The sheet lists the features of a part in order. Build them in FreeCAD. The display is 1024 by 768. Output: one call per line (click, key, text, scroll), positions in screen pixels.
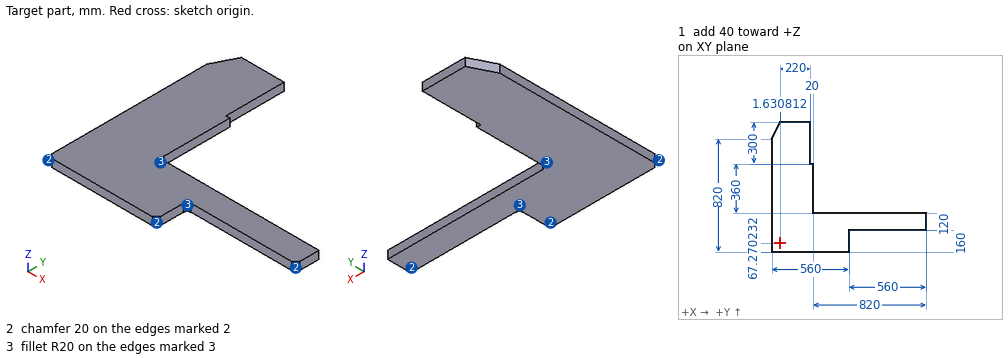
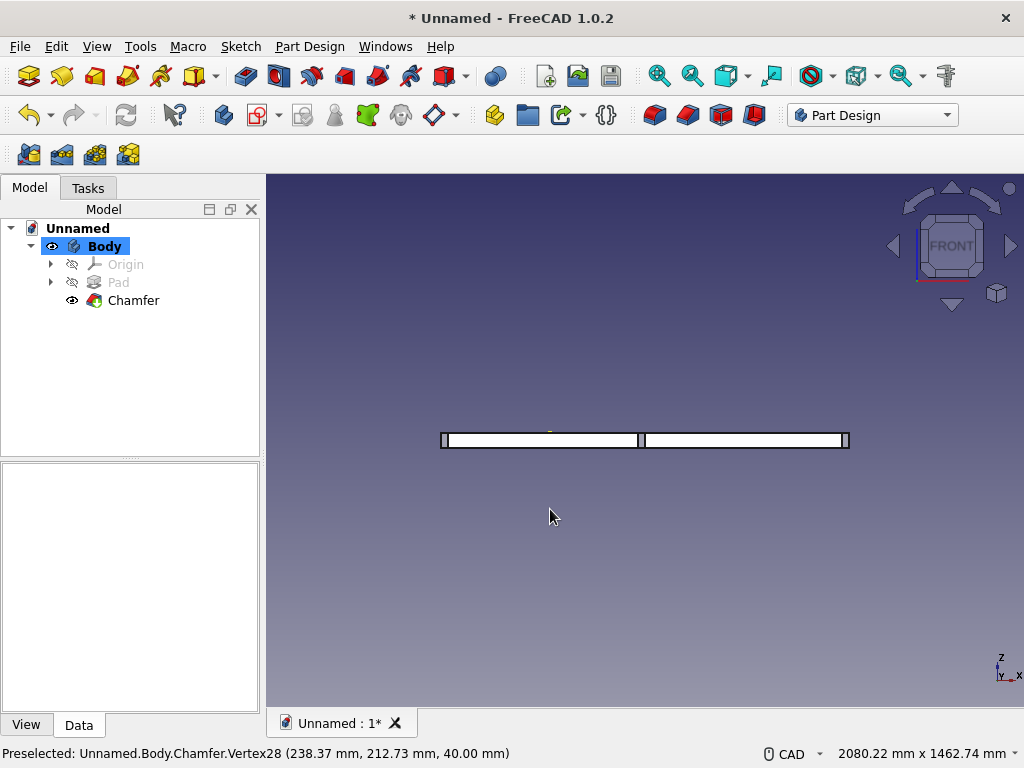
scroll(550, 439, up, 6)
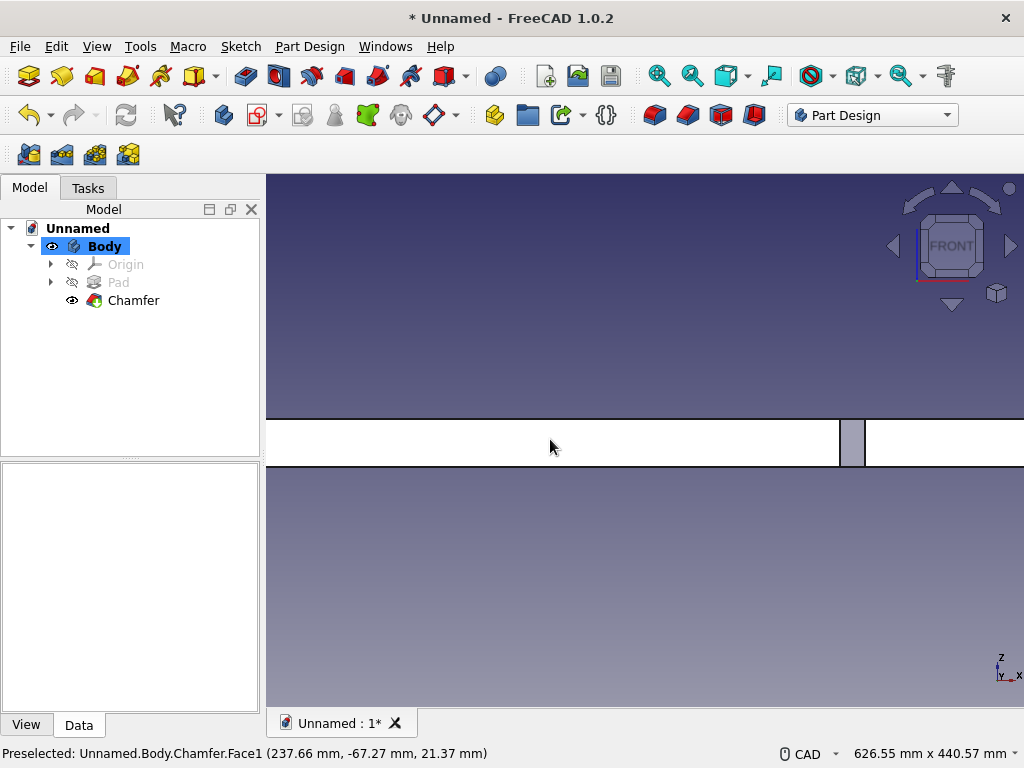
key(v)
key(f)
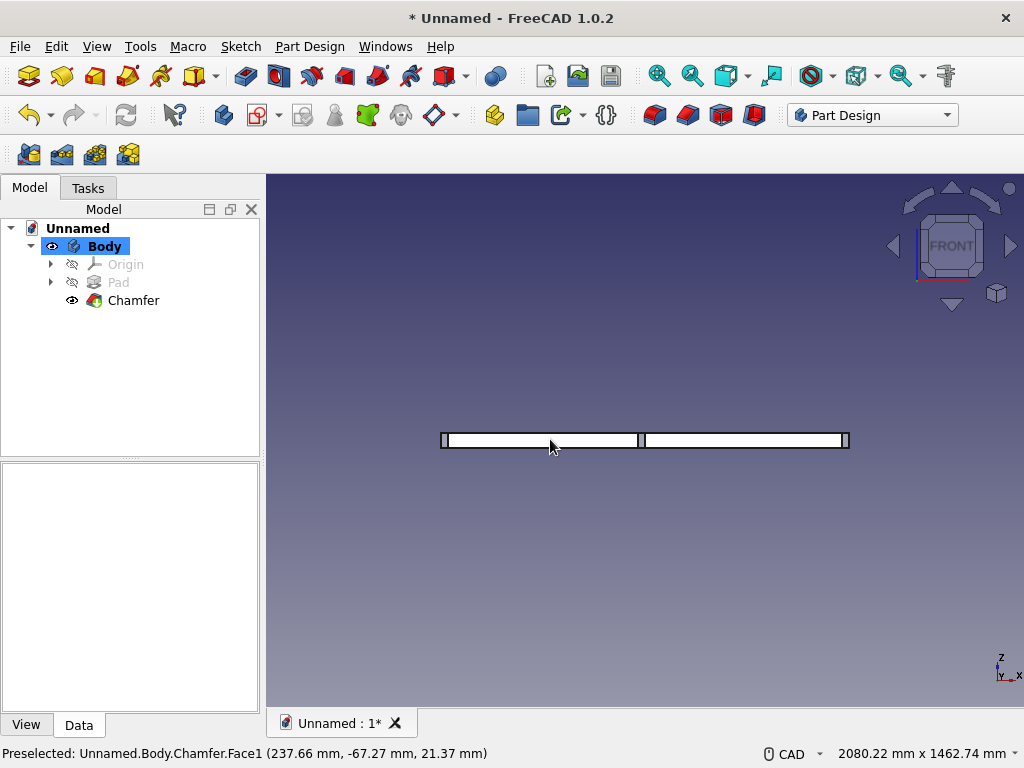
key(3)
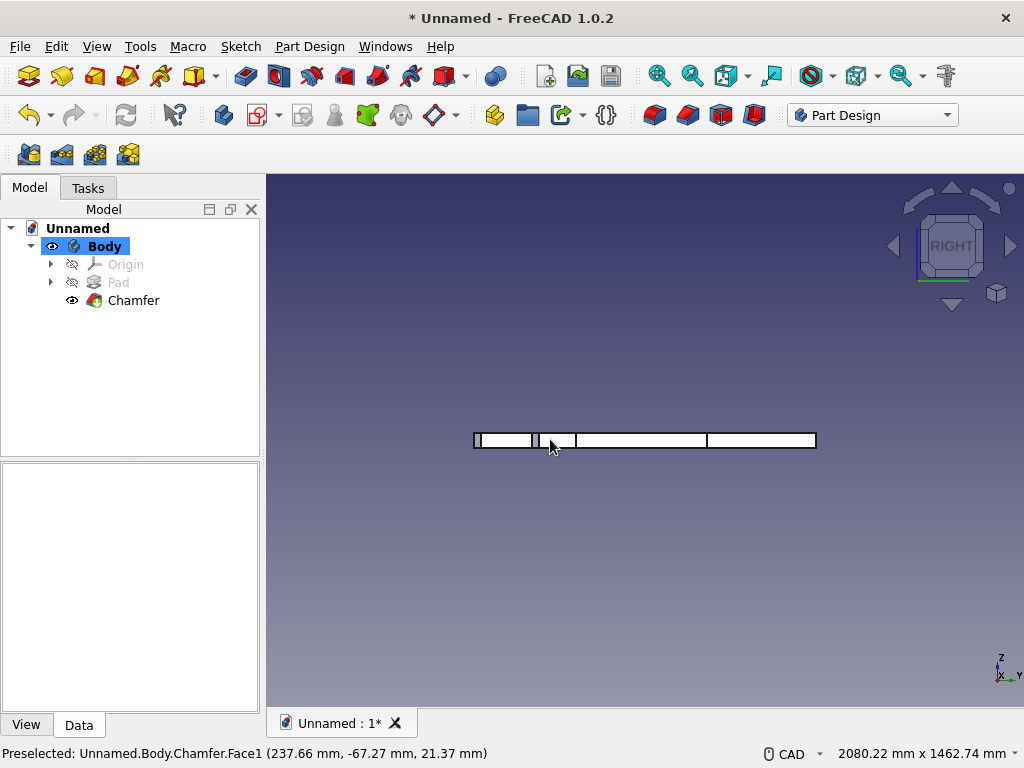
scroll(576, 439, up, 6)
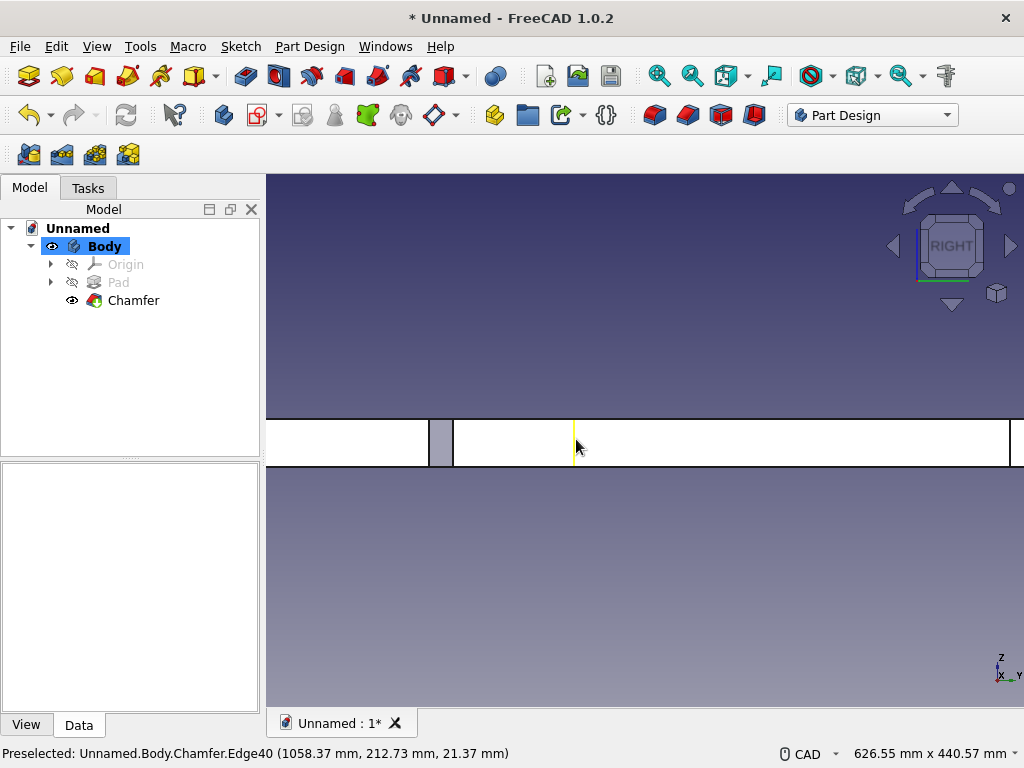
key(v)
key(f)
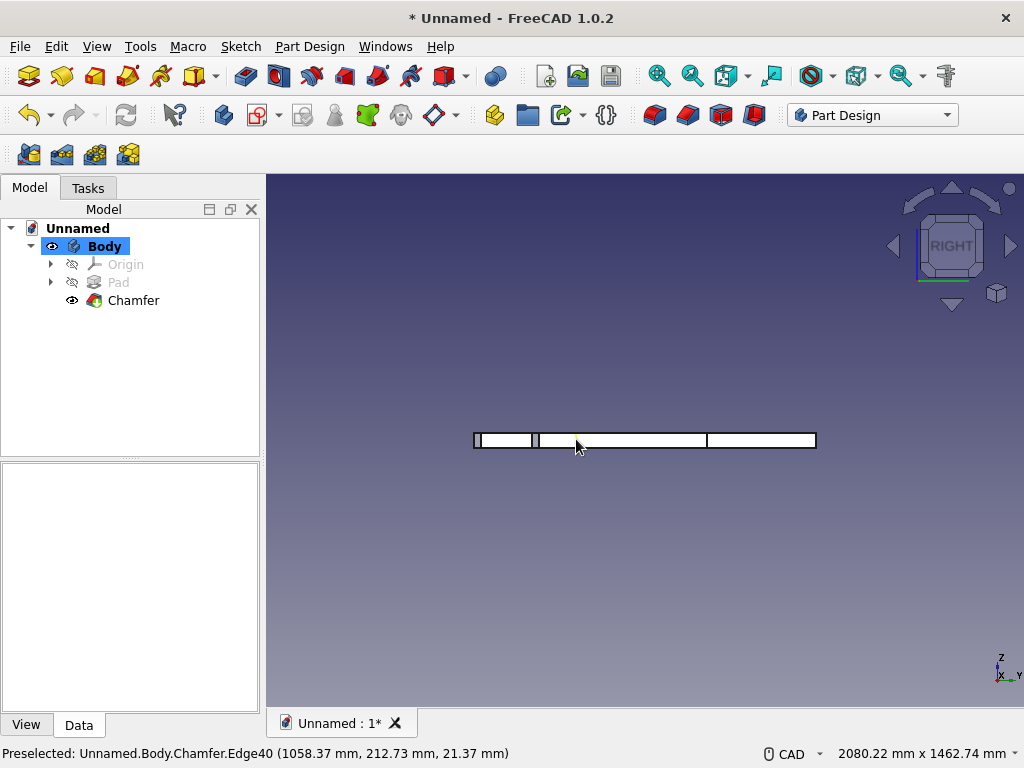
key(5)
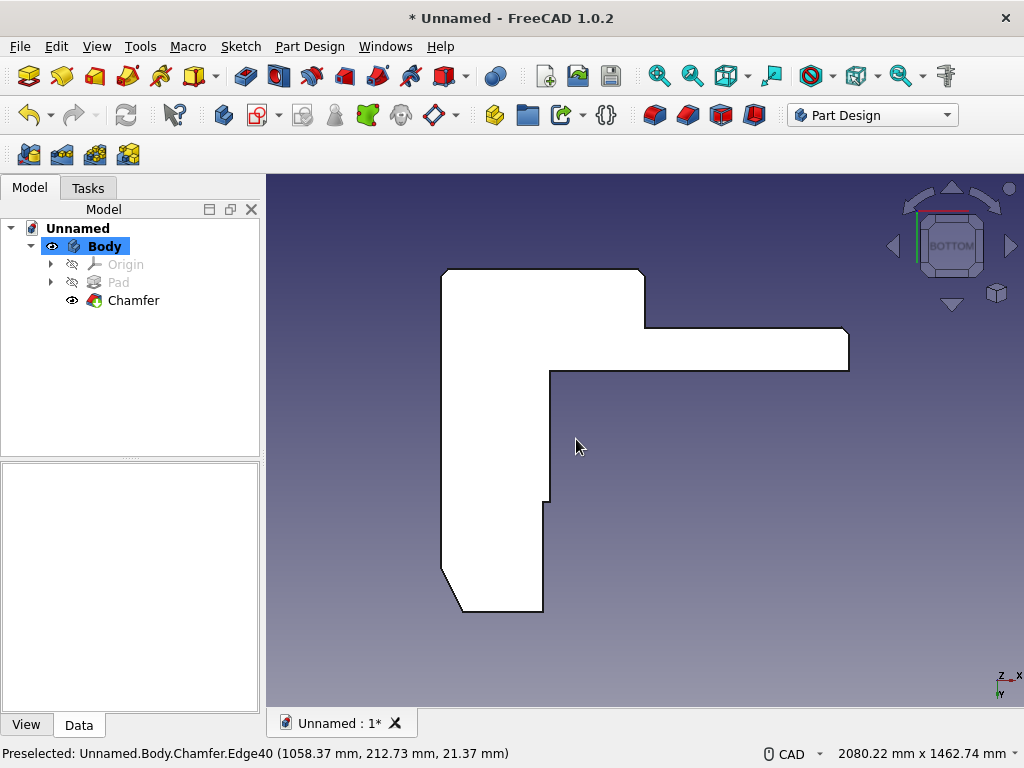
scroll(550, 370, up, 6)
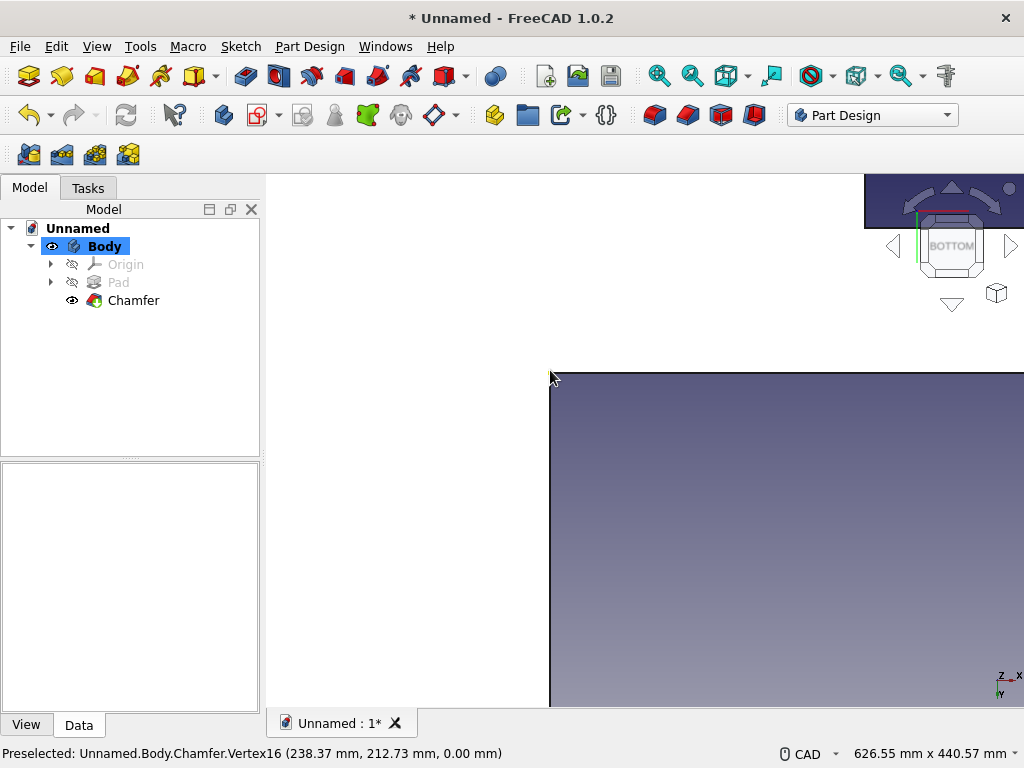
click(660, 76)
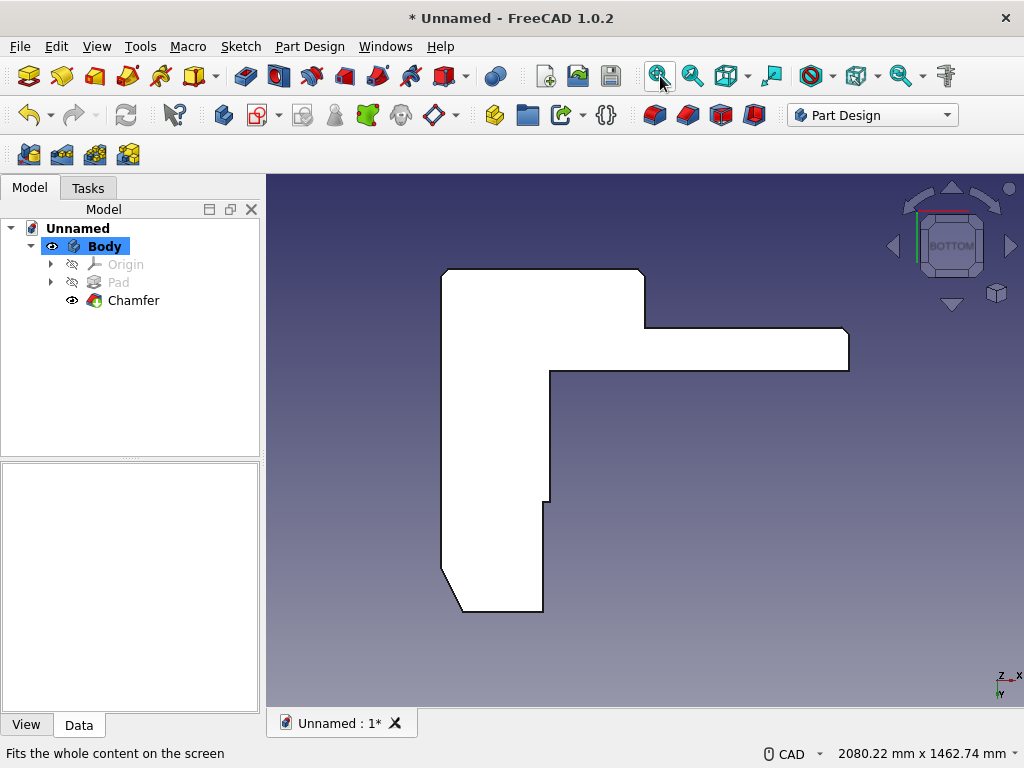
key(4)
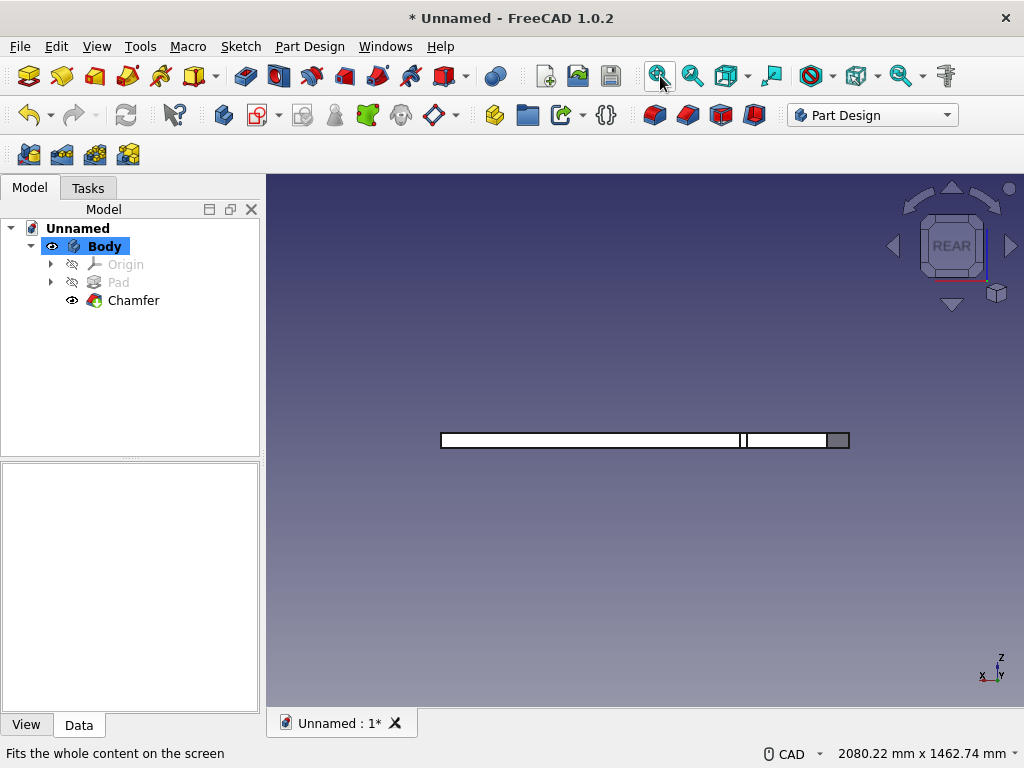
scroll(740, 439, up, 6)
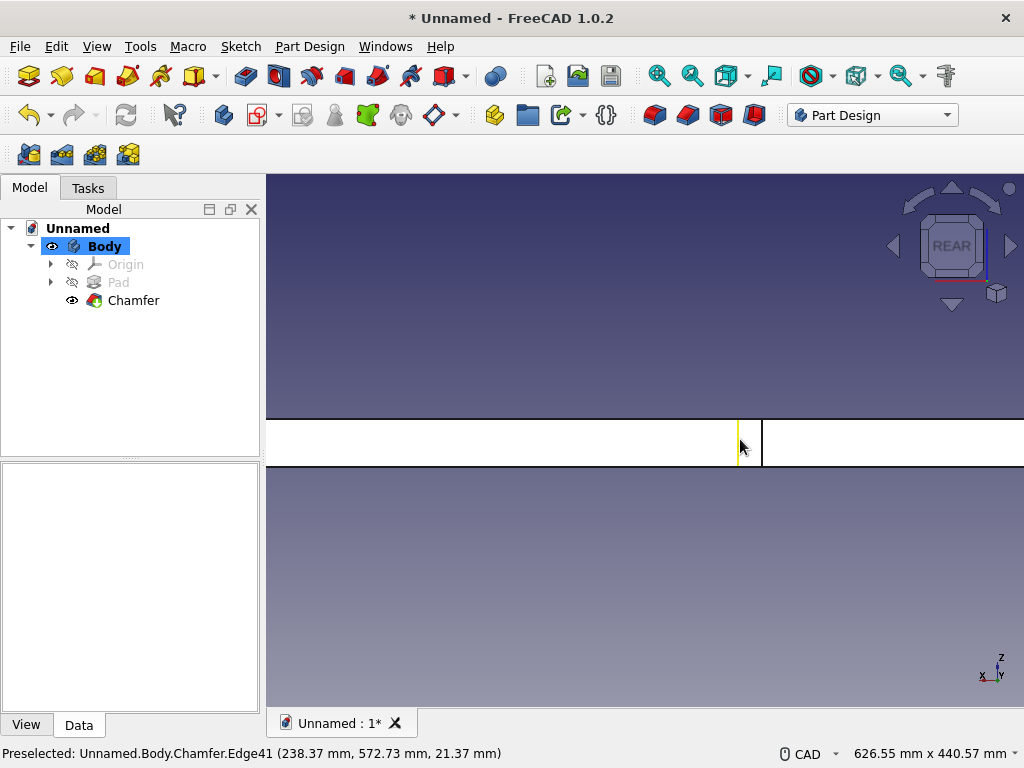
key(v)
key(f)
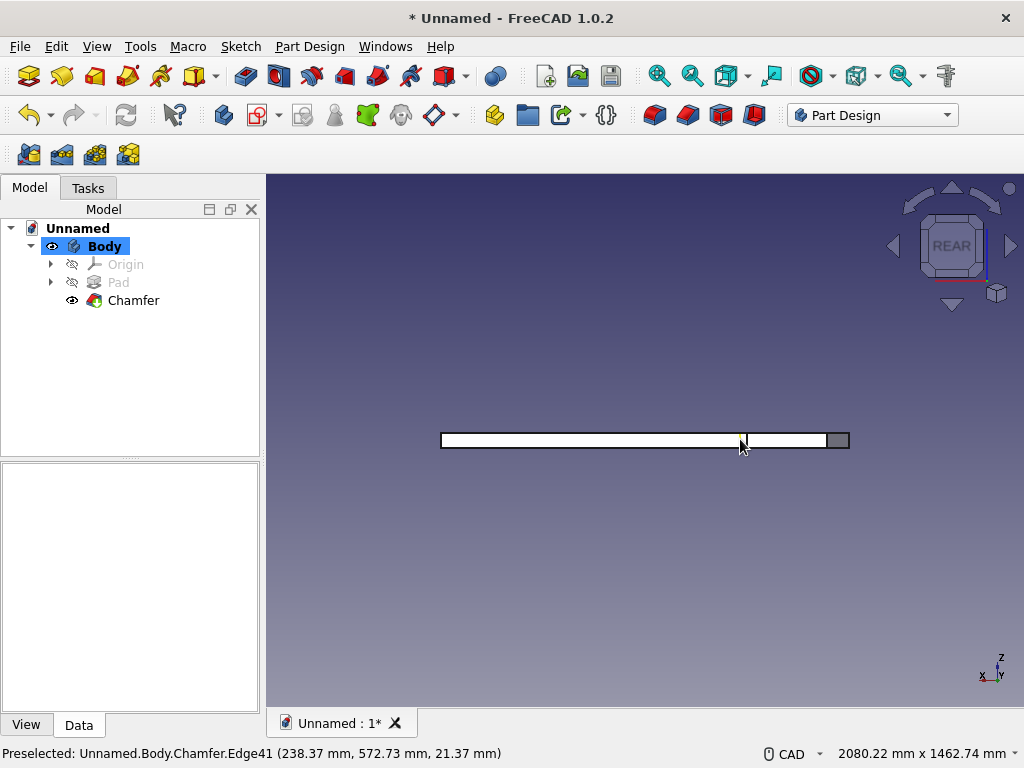
key(6)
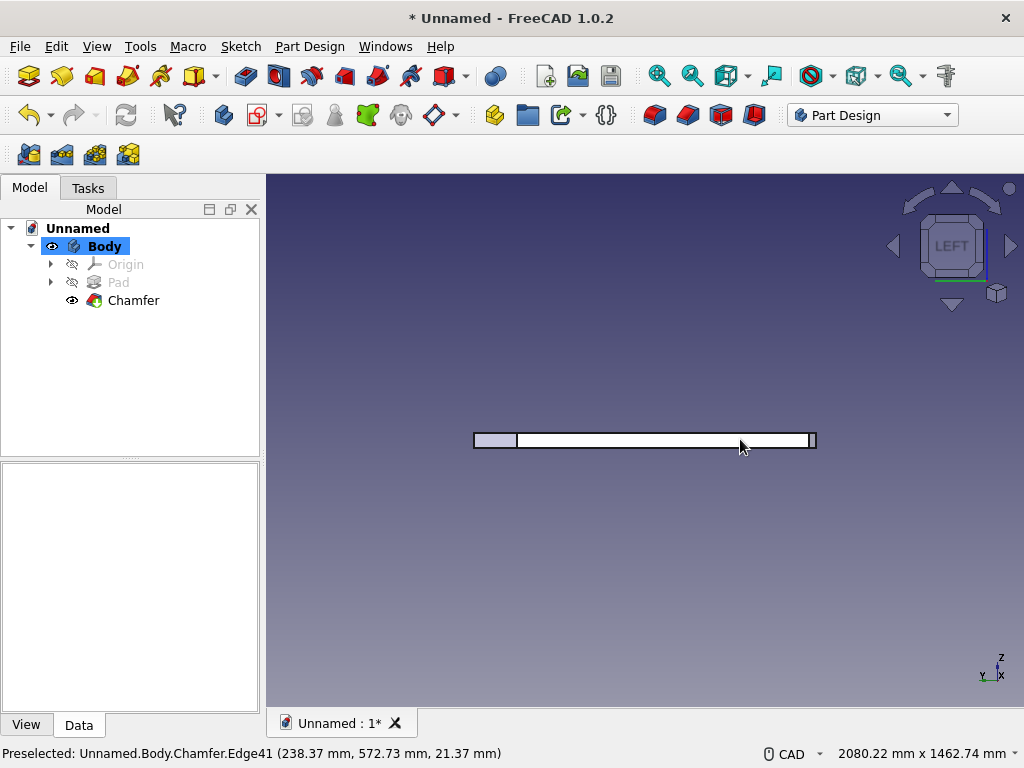
scroll(714, 439, up, 6)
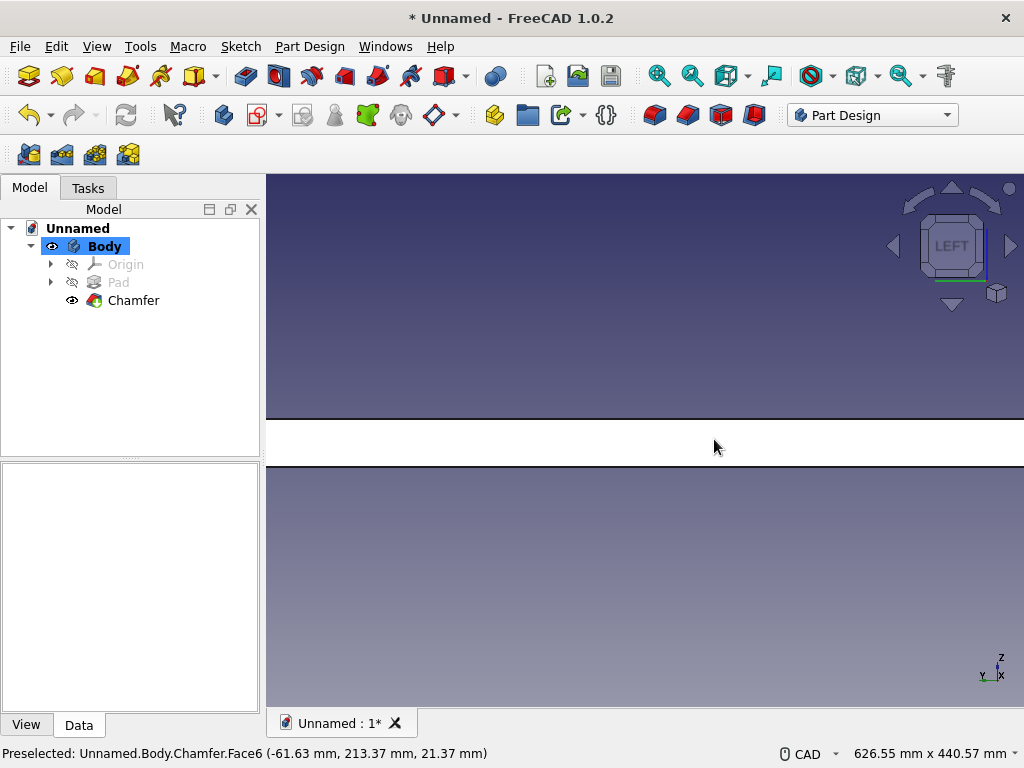
key(v)
key(f)